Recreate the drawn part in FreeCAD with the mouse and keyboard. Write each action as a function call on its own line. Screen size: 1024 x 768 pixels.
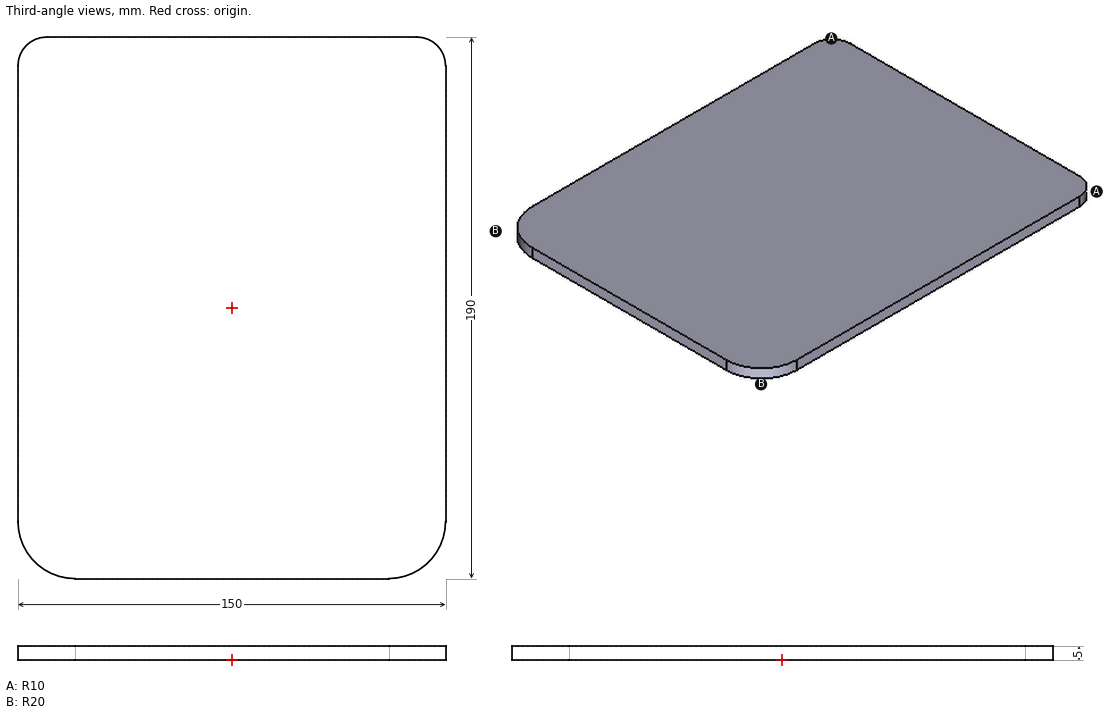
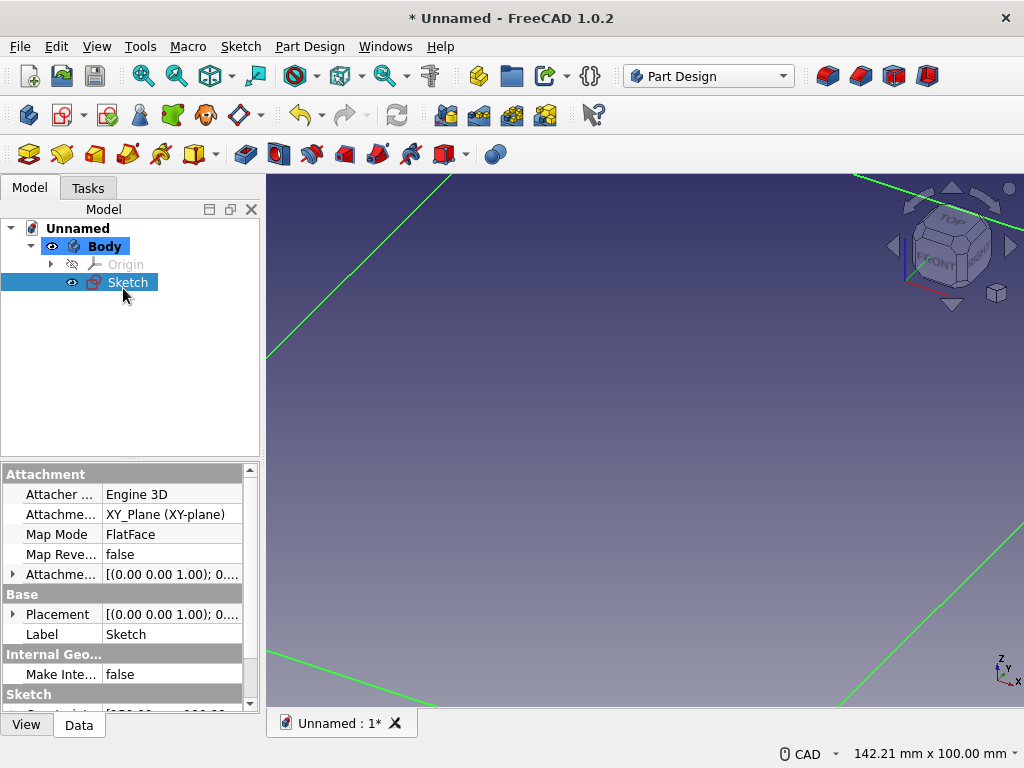
click(29, 154)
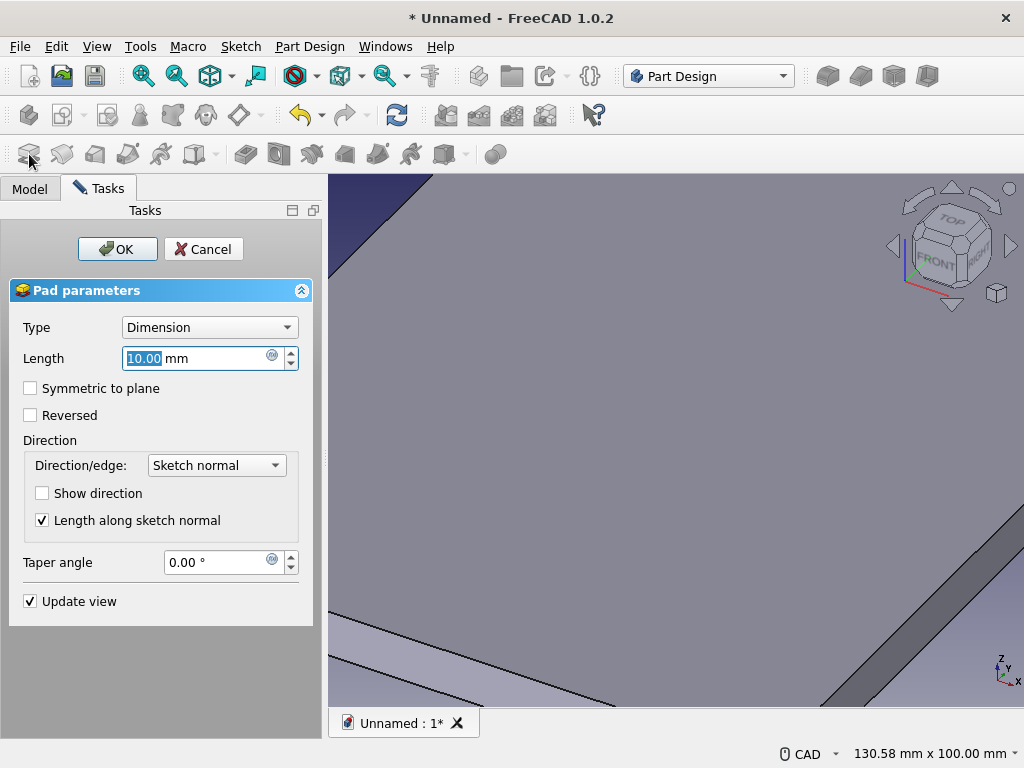
text(5)
key(Tab)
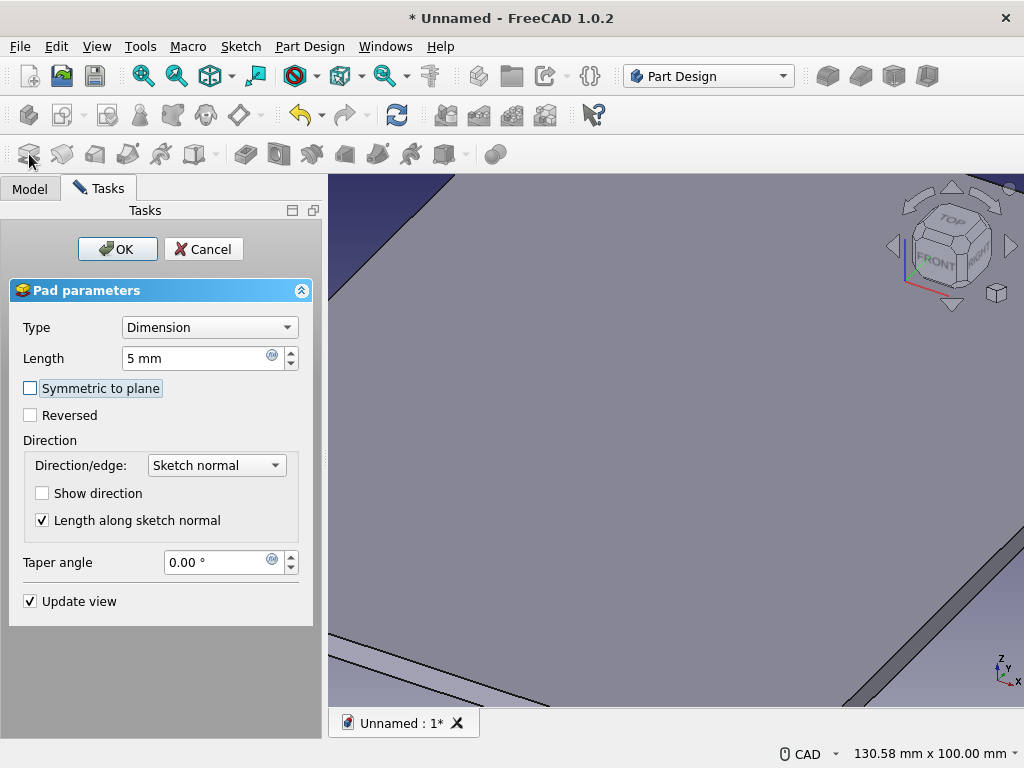
click(118, 249)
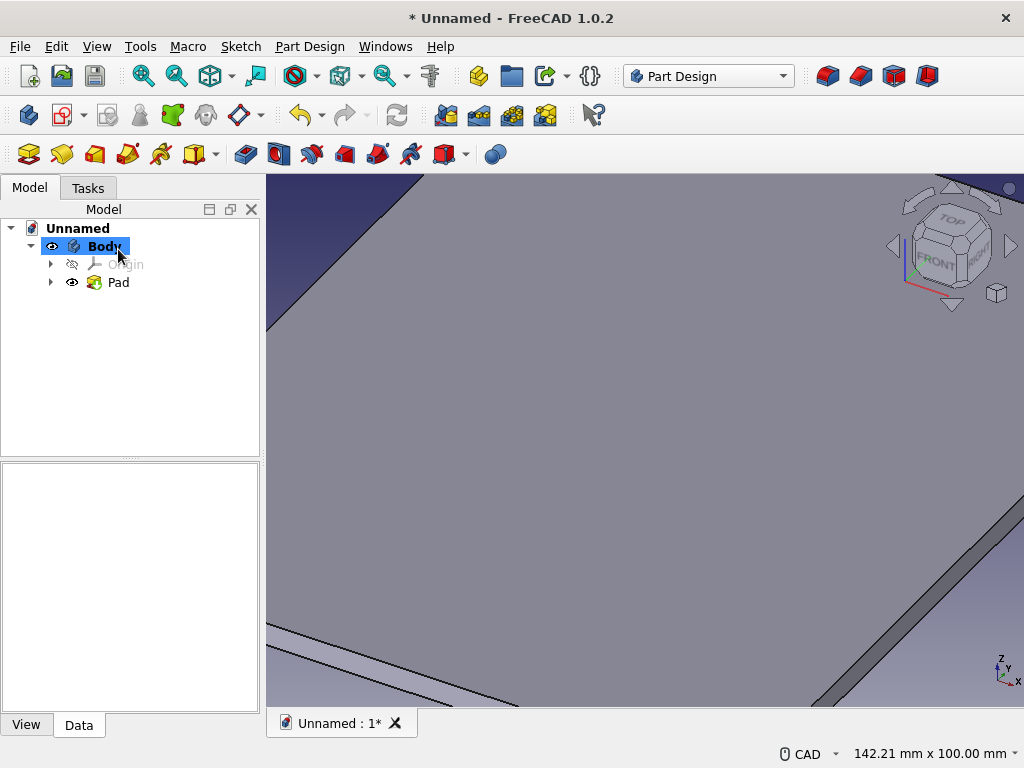
click(144, 76)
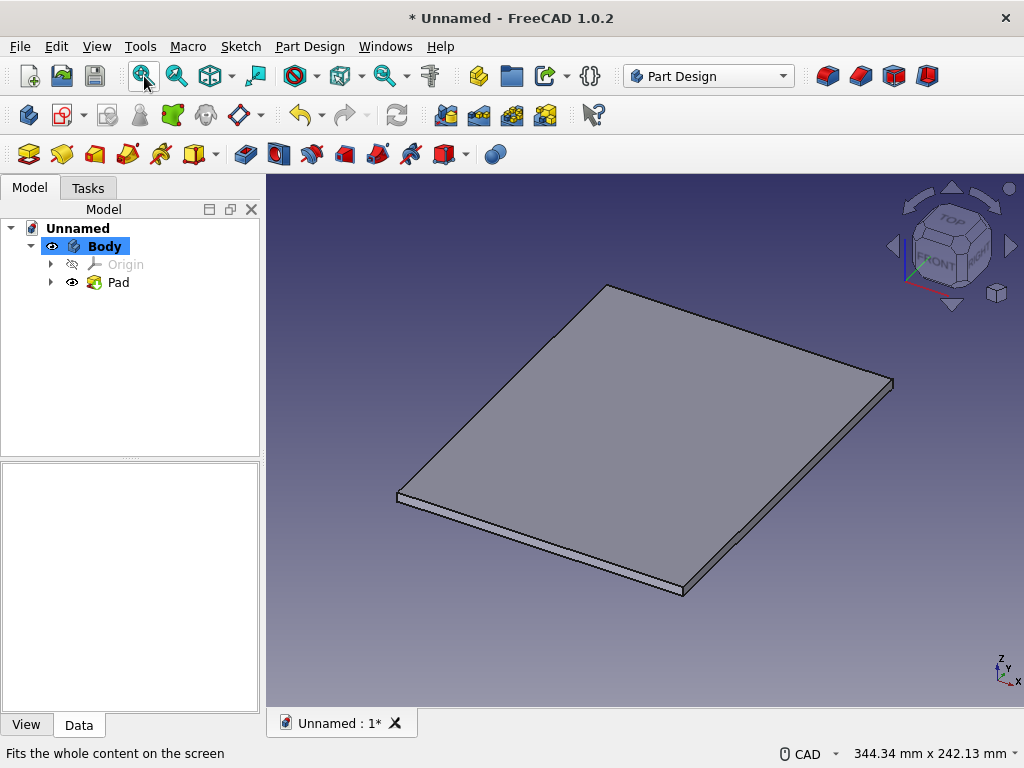
scroll(607, 288, up, 7)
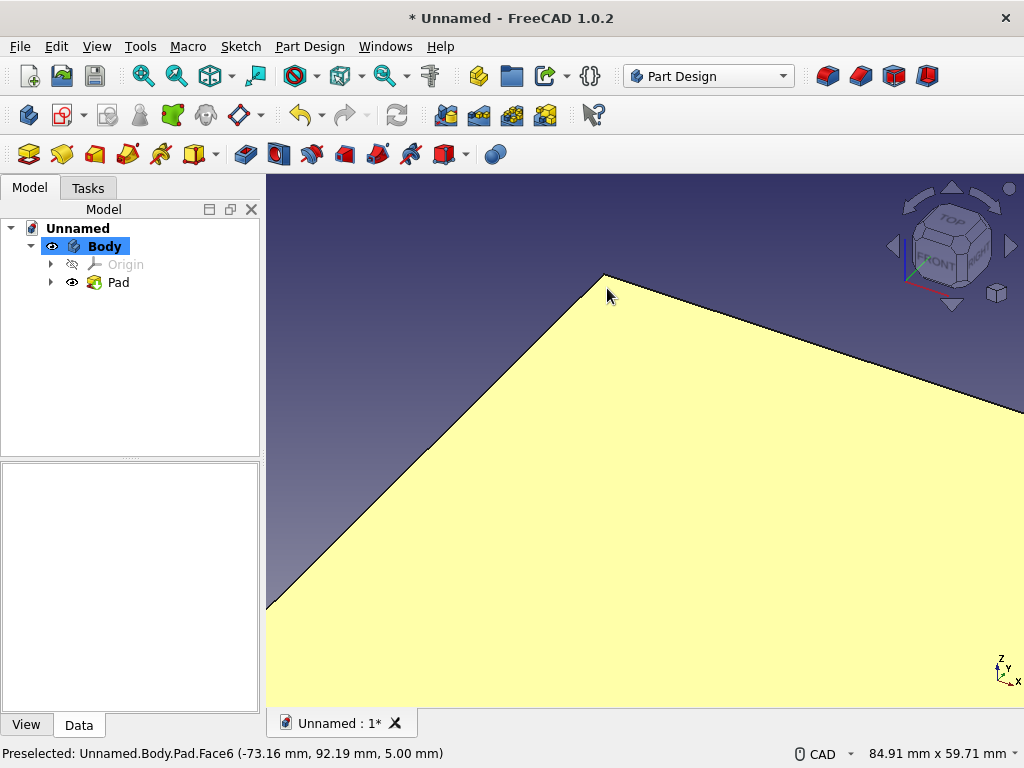
click(144, 76)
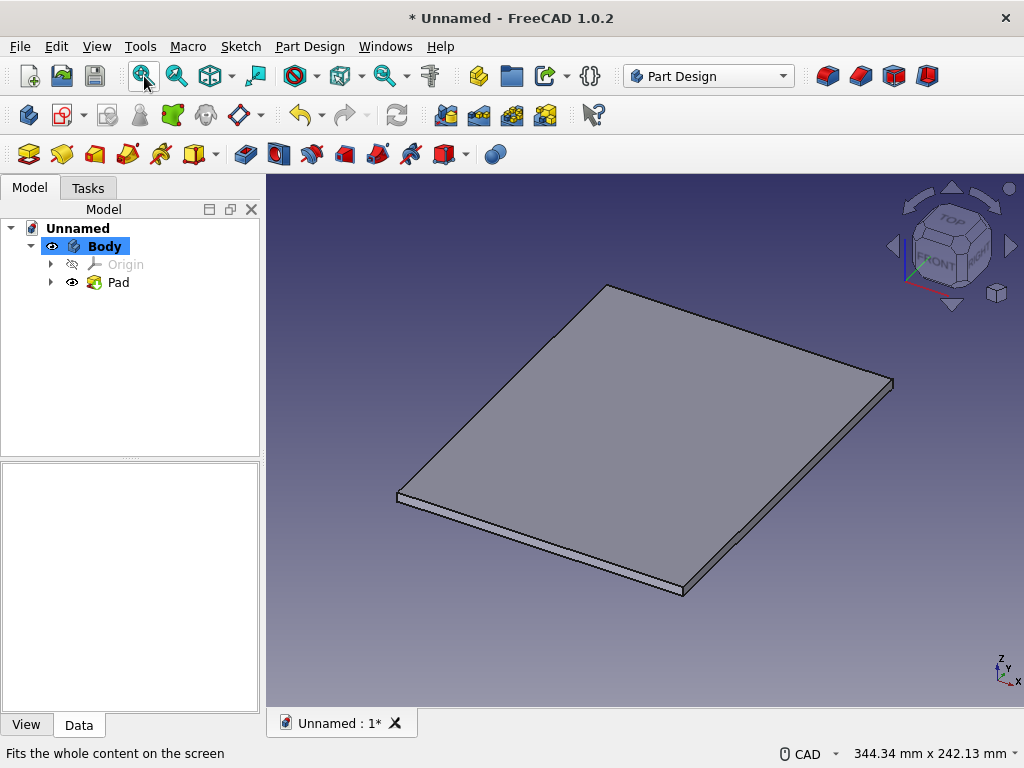
key(0)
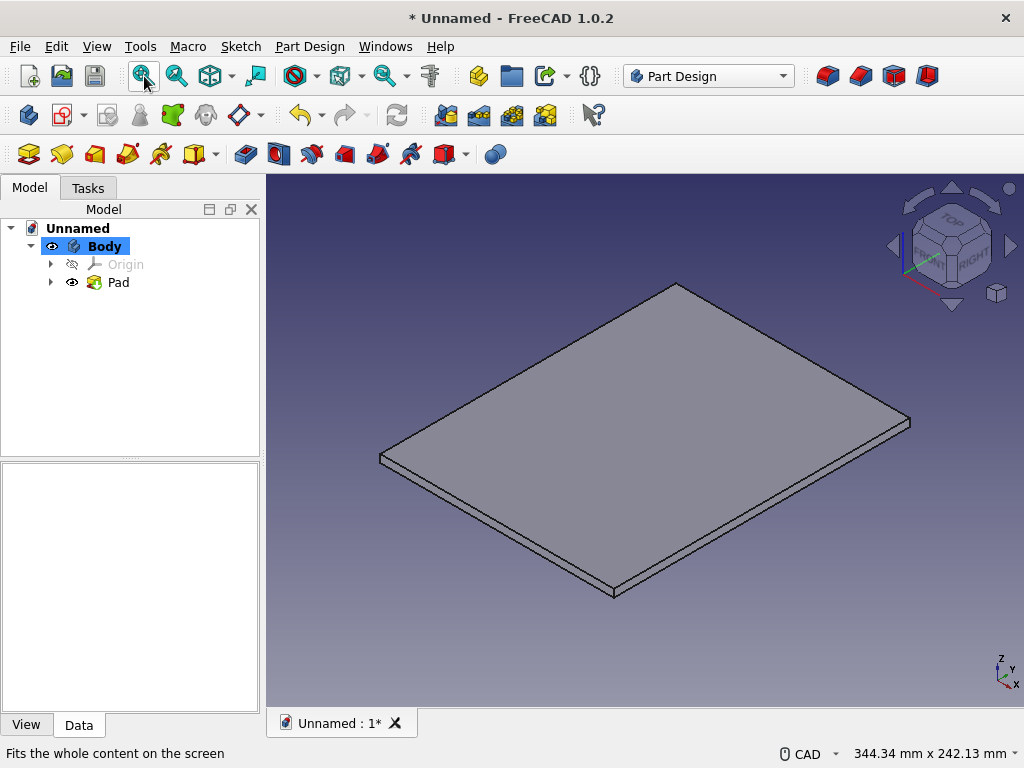
scroll(676, 287, up, 7)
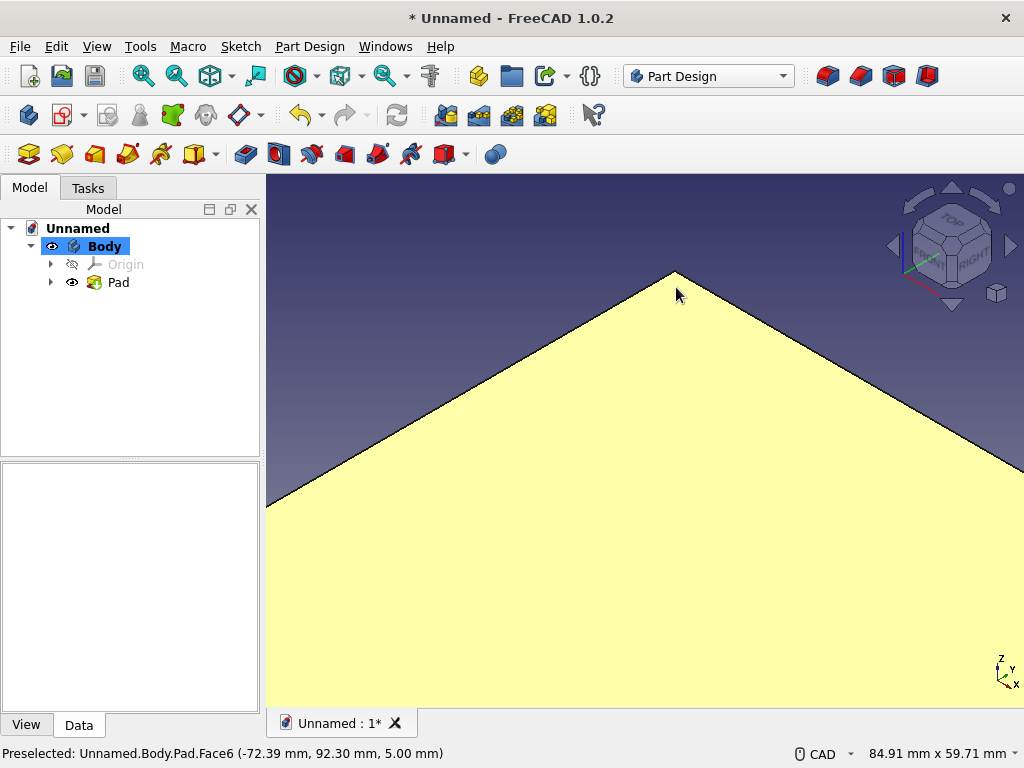
click(144, 76)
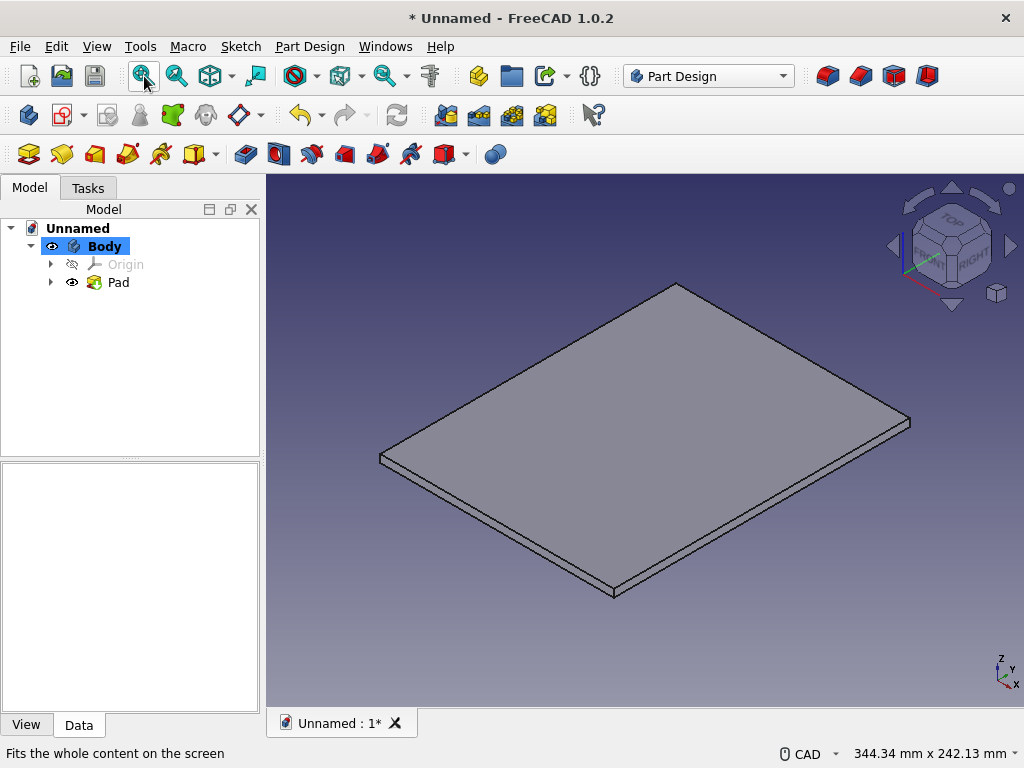
key(2)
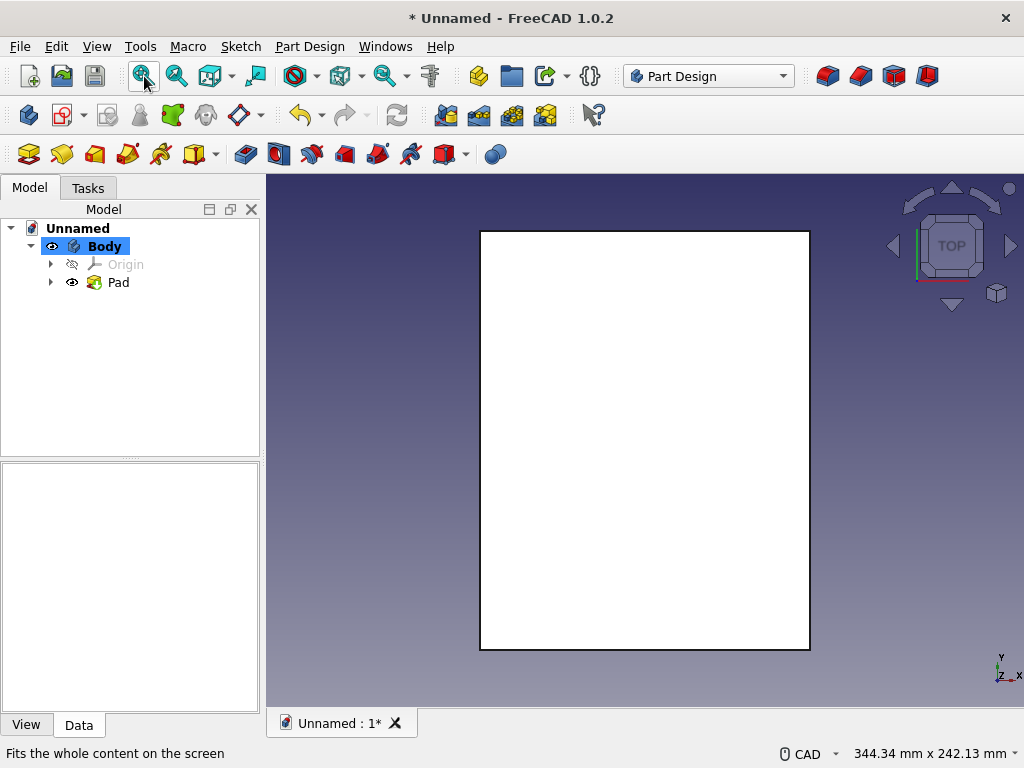
scroll(480, 230, up, 7)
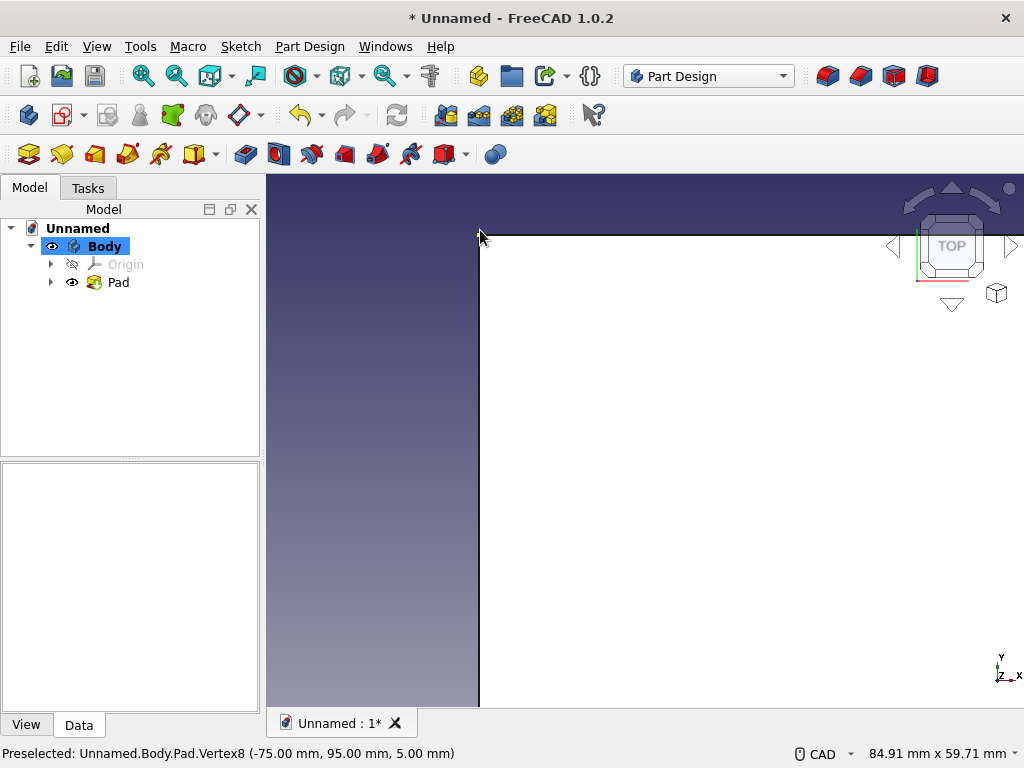
click(144, 76)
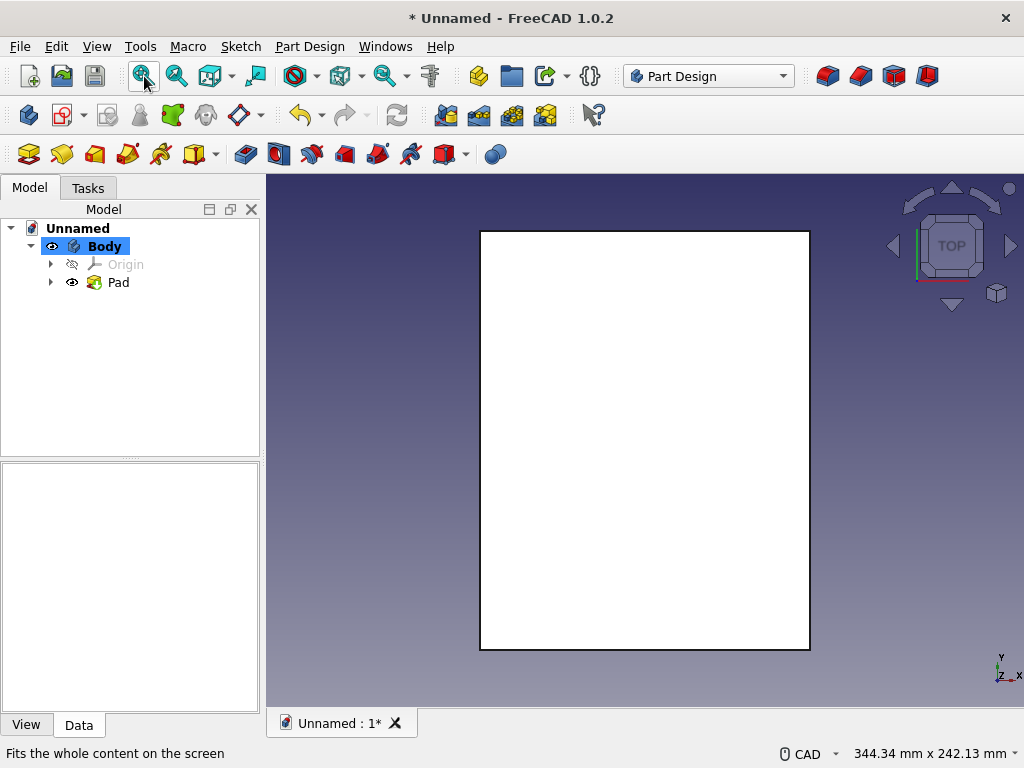
key(1)